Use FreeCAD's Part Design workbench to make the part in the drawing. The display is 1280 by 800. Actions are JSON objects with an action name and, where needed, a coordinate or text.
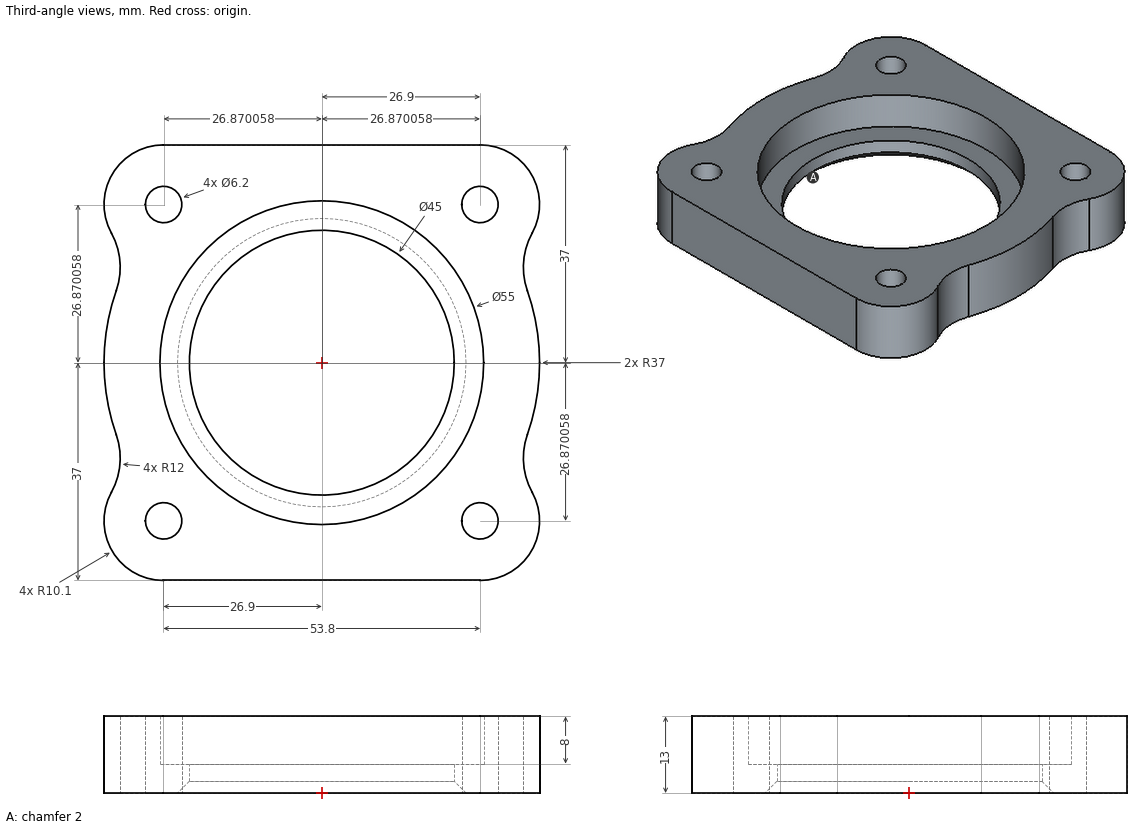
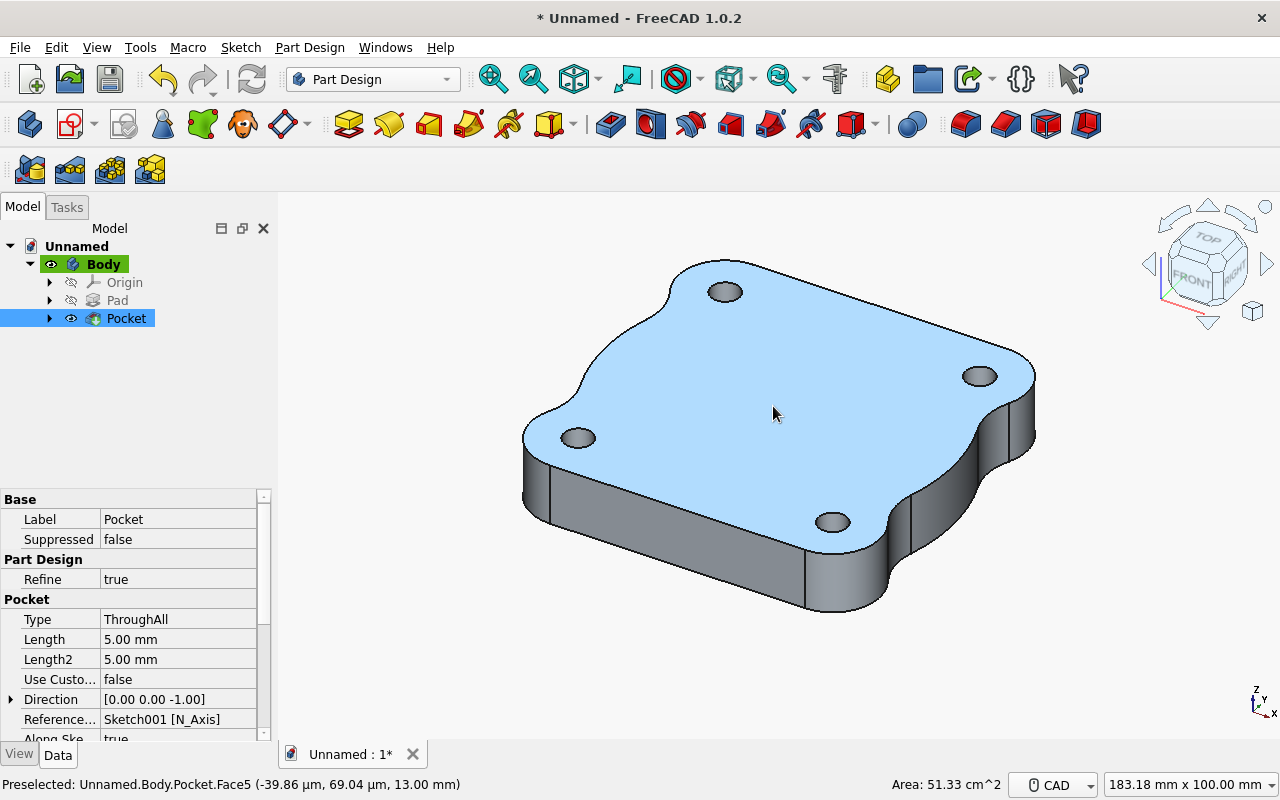
{"action": "left_click", "coordinate": [70, 124]}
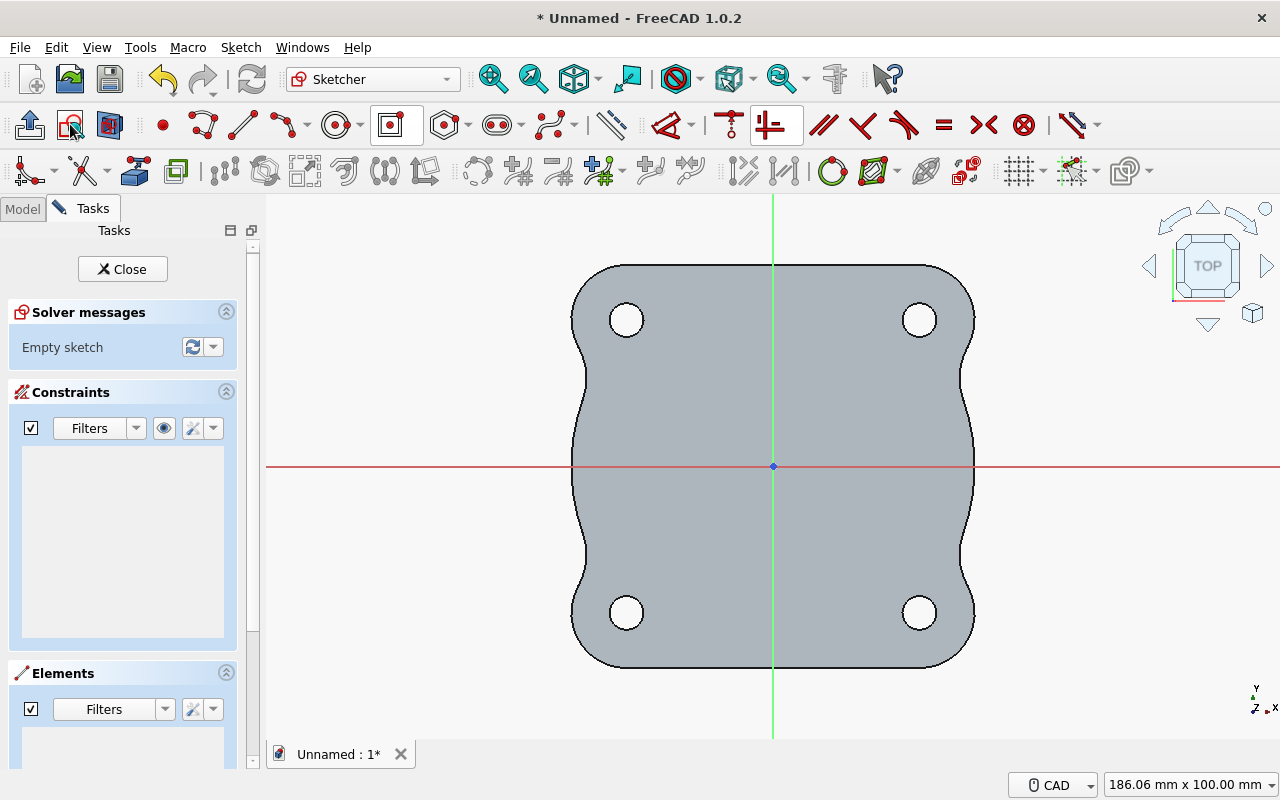
{"action": "left_click", "coordinate": [336, 126]}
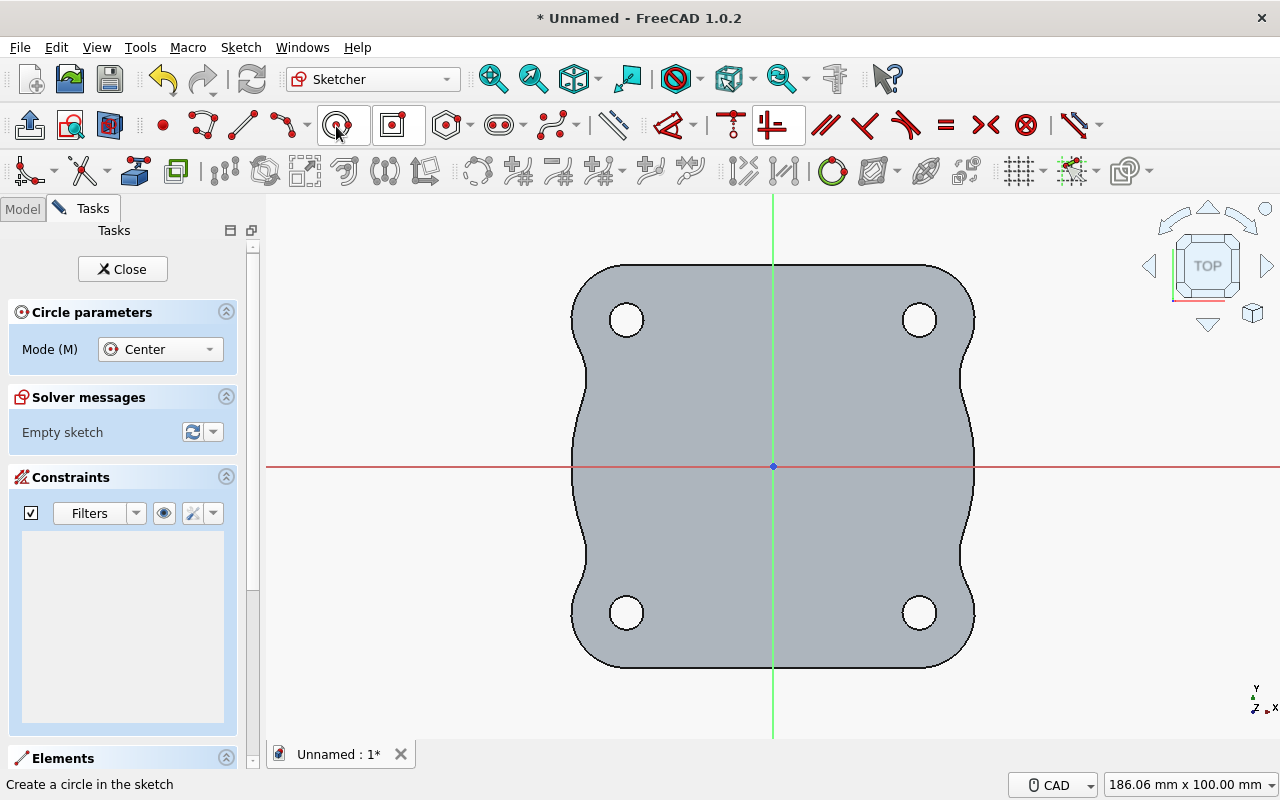
{"action": "left_click", "coordinate": [773, 466]}
{"action": "left_click", "coordinate": [879, 361]}
{"action": "key", "text": "Escape"}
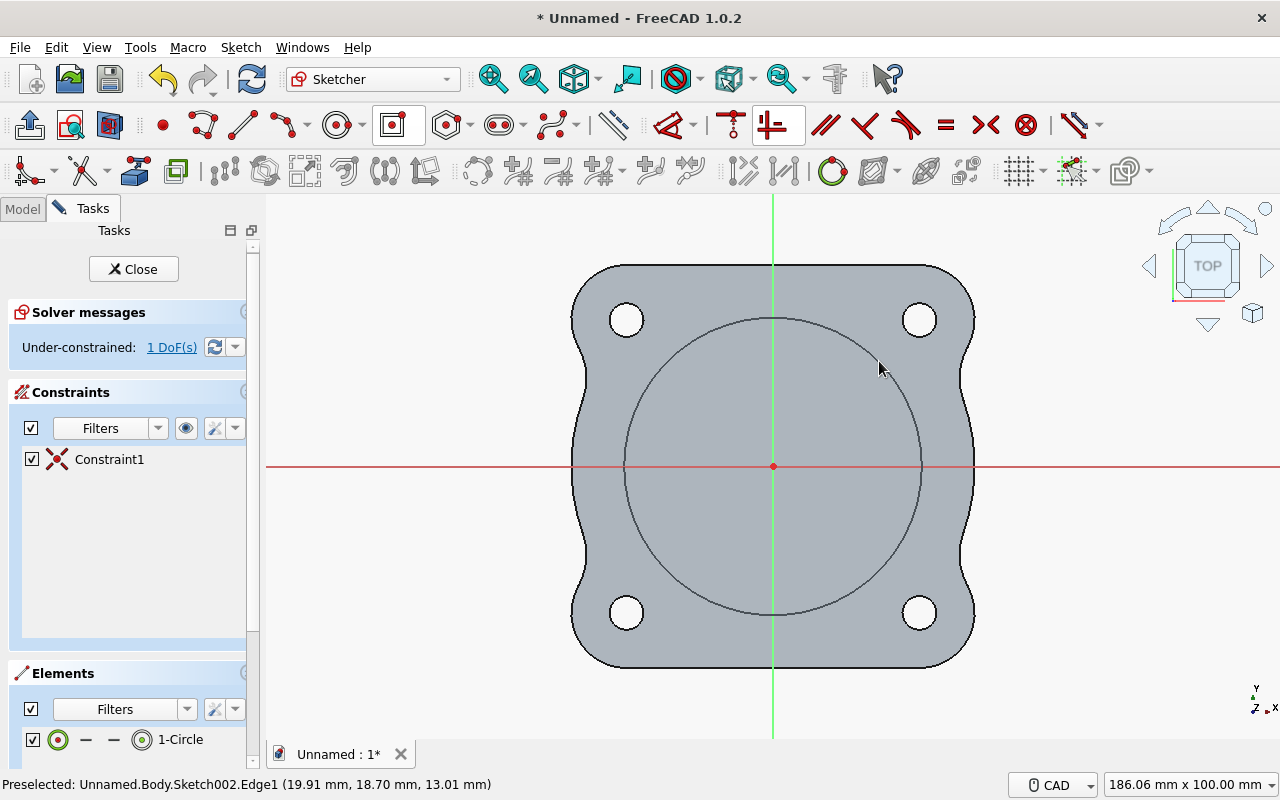
{"action": "left_click", "coordinate": [668, 126]}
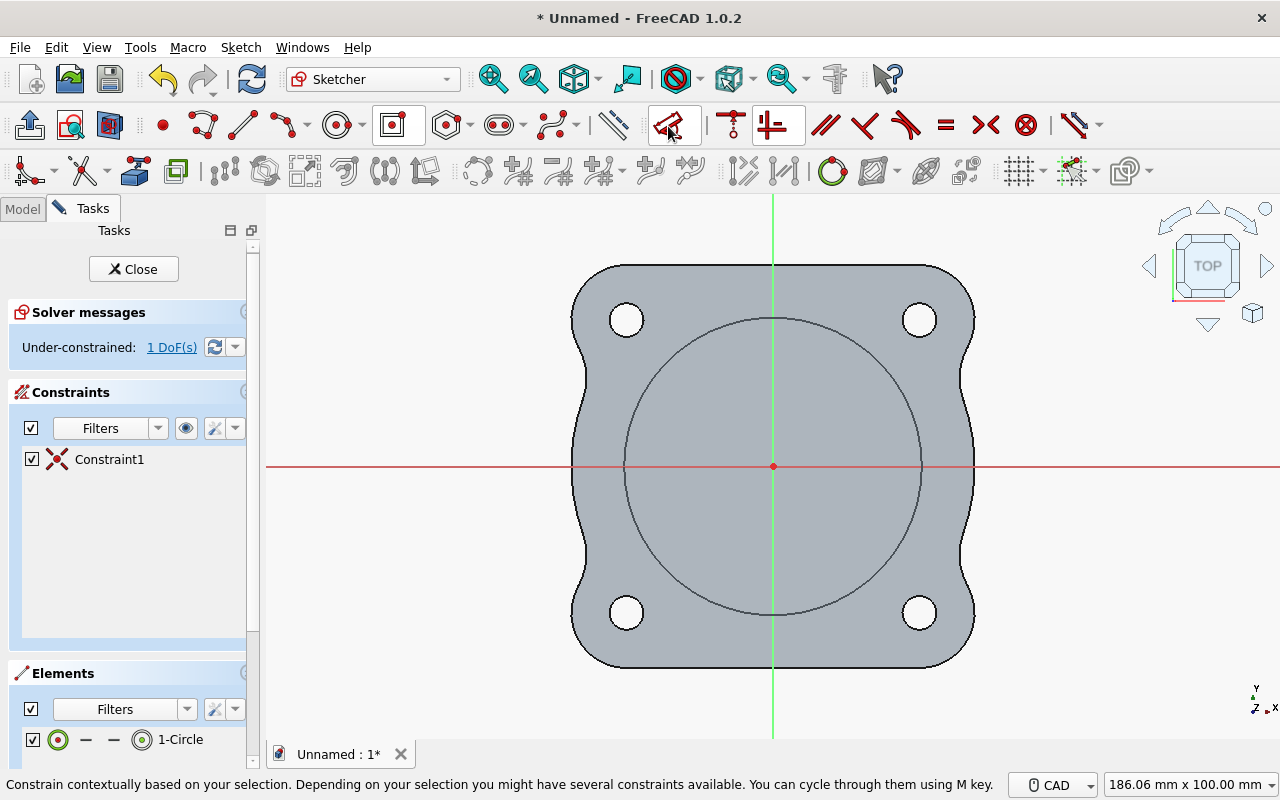
{"action": "left_click", "coordinate": [878, 361]}
{"action": "left_click", "coordinate": [901, 338]}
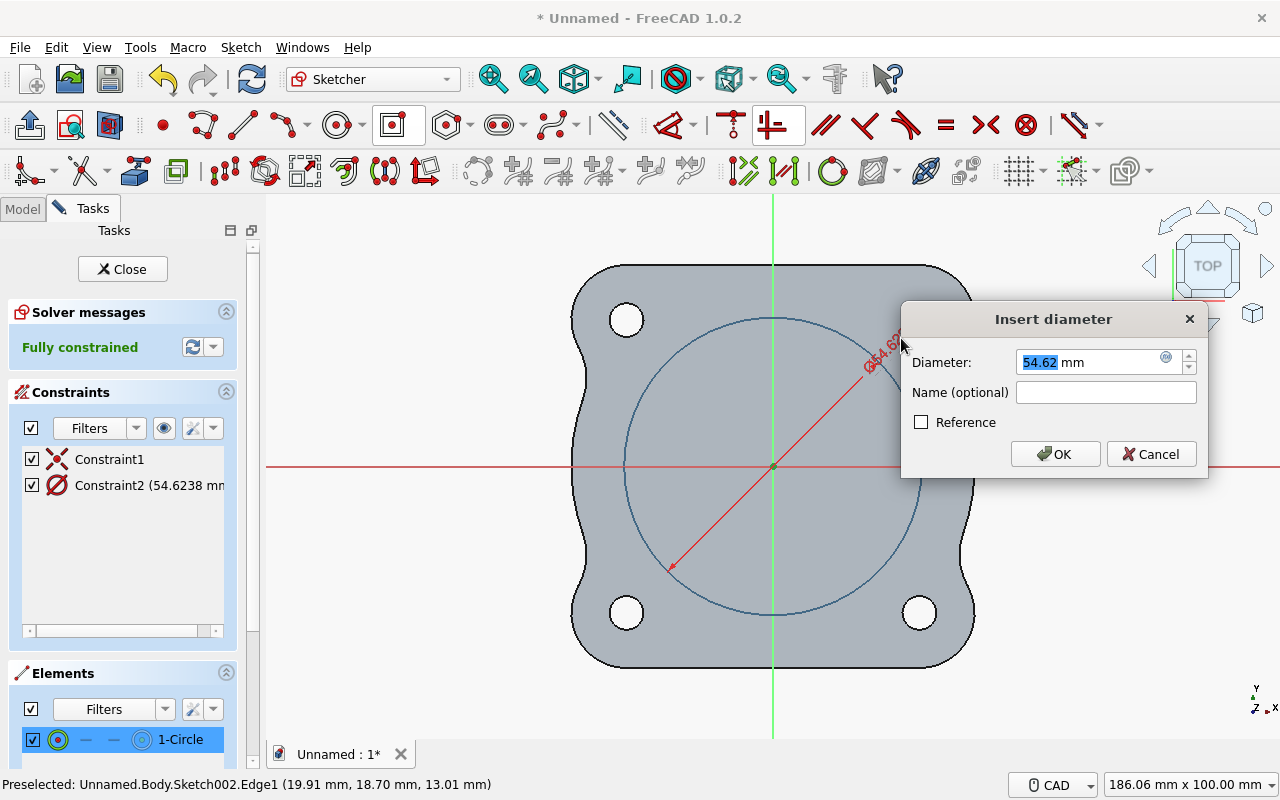
{"action": "type", "text": "55"}
{"action": "key", "text": "Return"}
{"action": "key", "text": "Escape"}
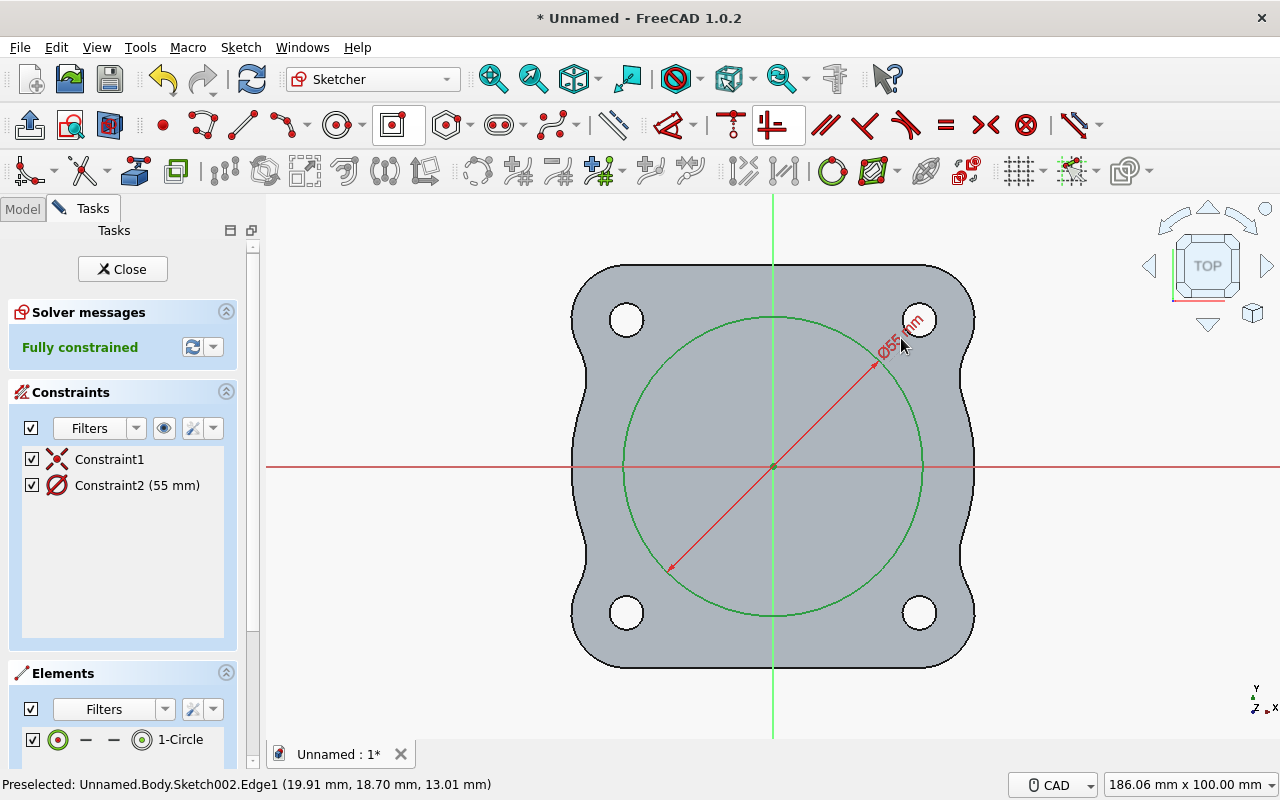
{"action": "left_click", "coordinate": [123, 269]}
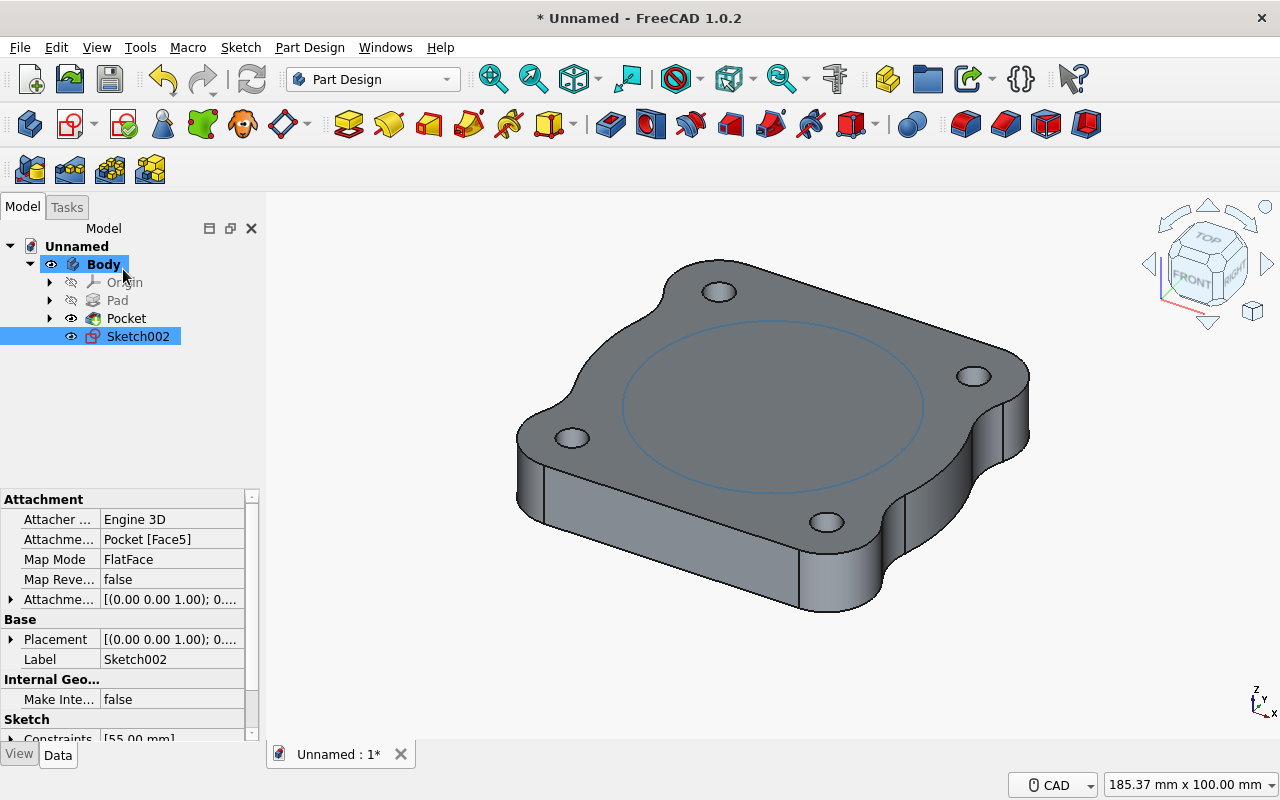
{"action": "left_click", "coordinate": [612, 124]}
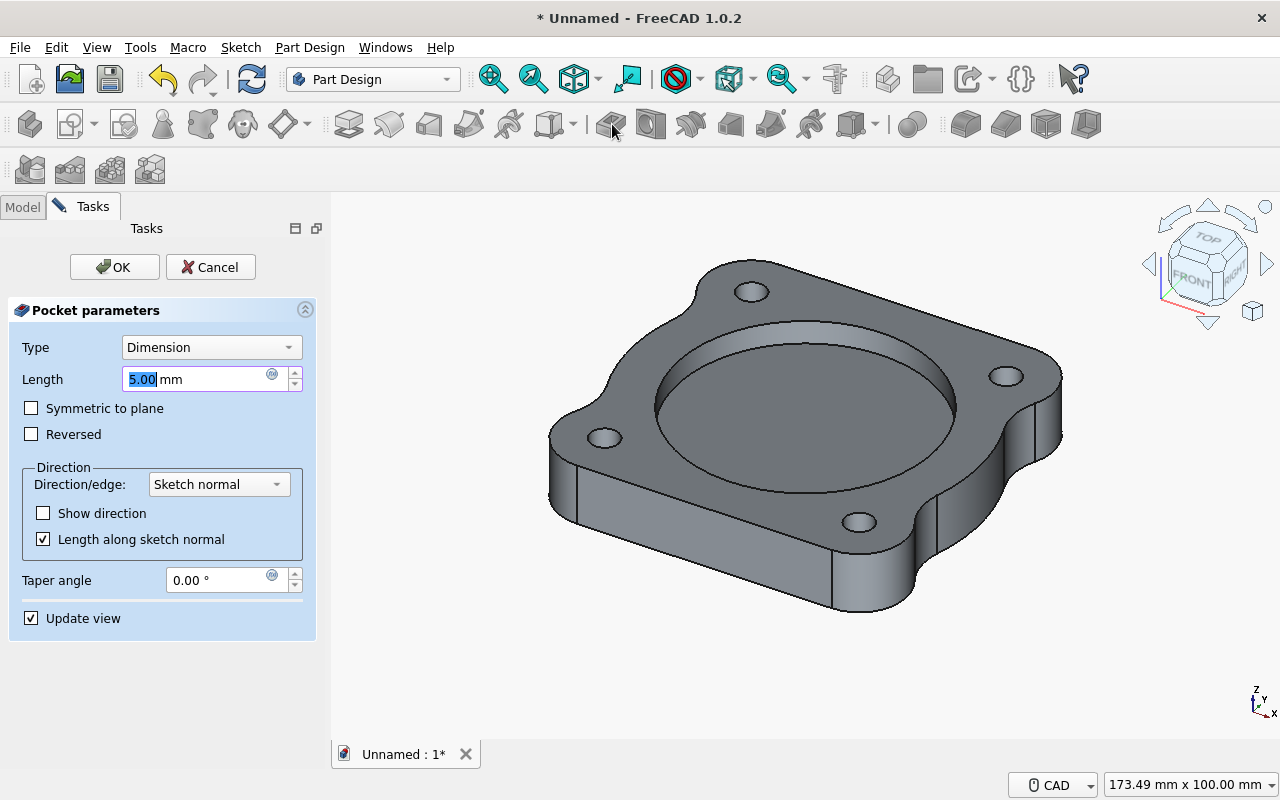
{"action": "type", "text": "8"}
{"action": "key", "text": "Tab"}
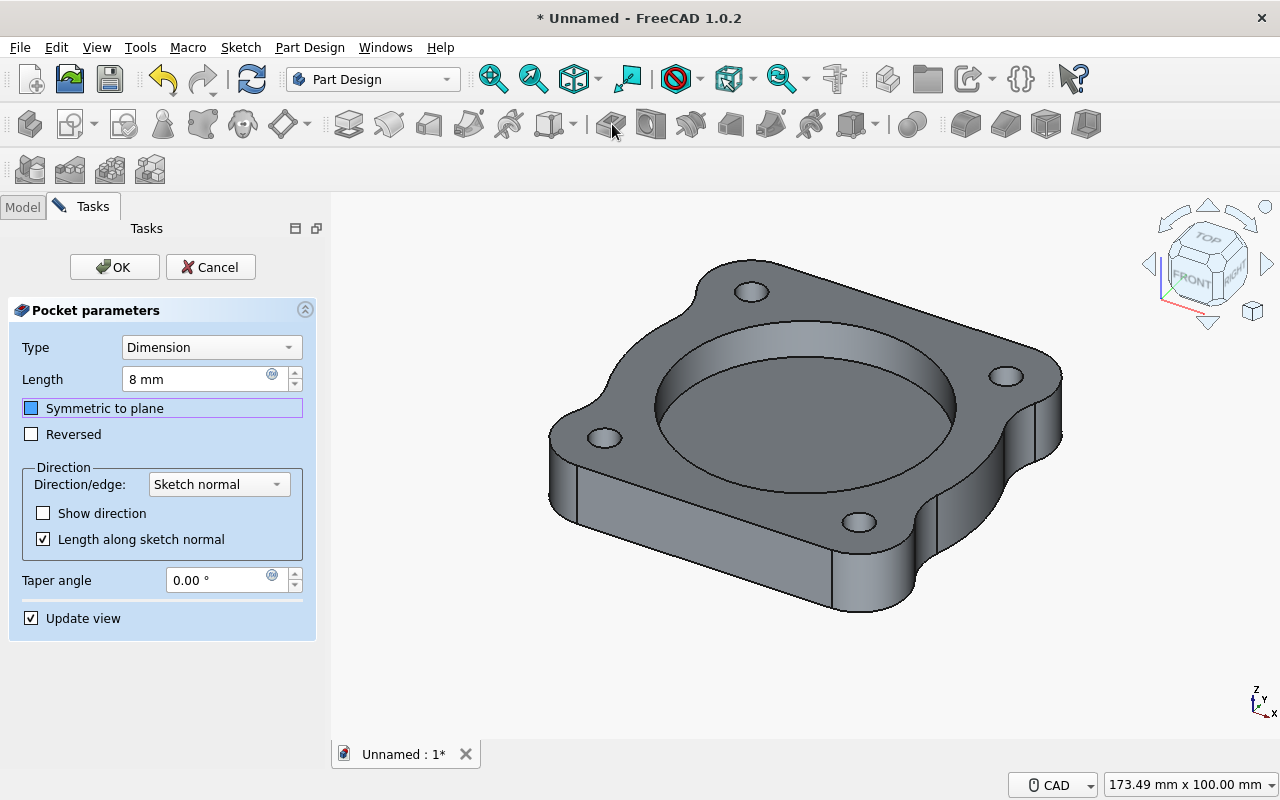
{"action": "left_click", "coordinate": [115, 267]}